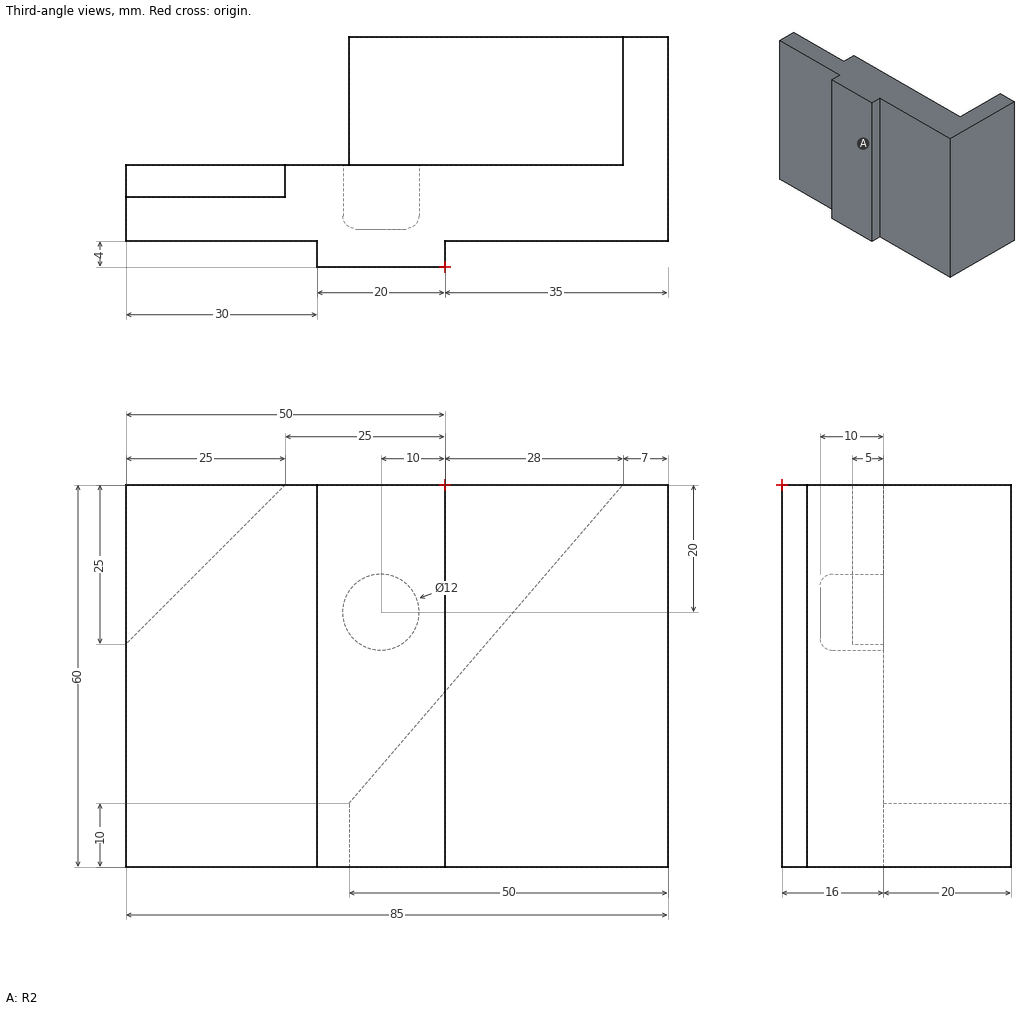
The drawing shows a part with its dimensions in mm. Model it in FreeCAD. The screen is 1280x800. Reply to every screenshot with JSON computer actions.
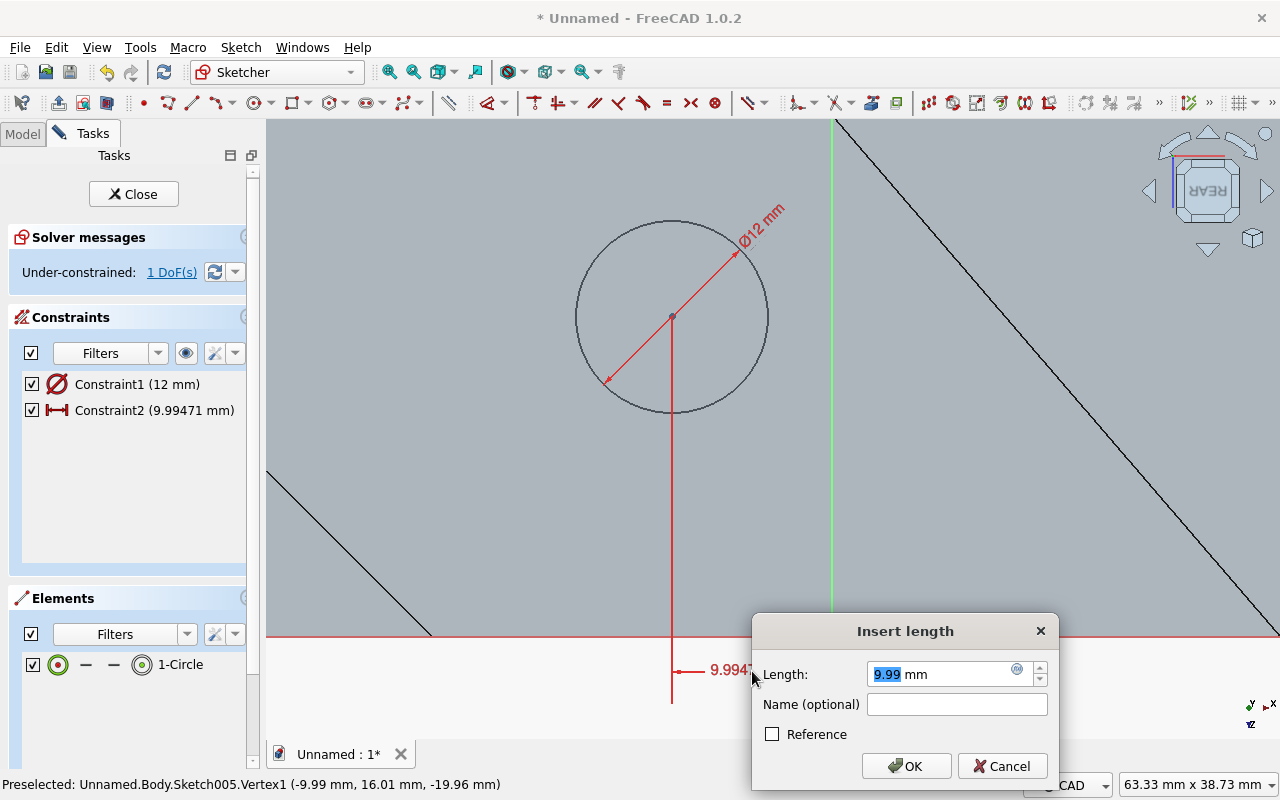
{"action": "type", "text": "10"}
{"action": "key", "text": "Return"}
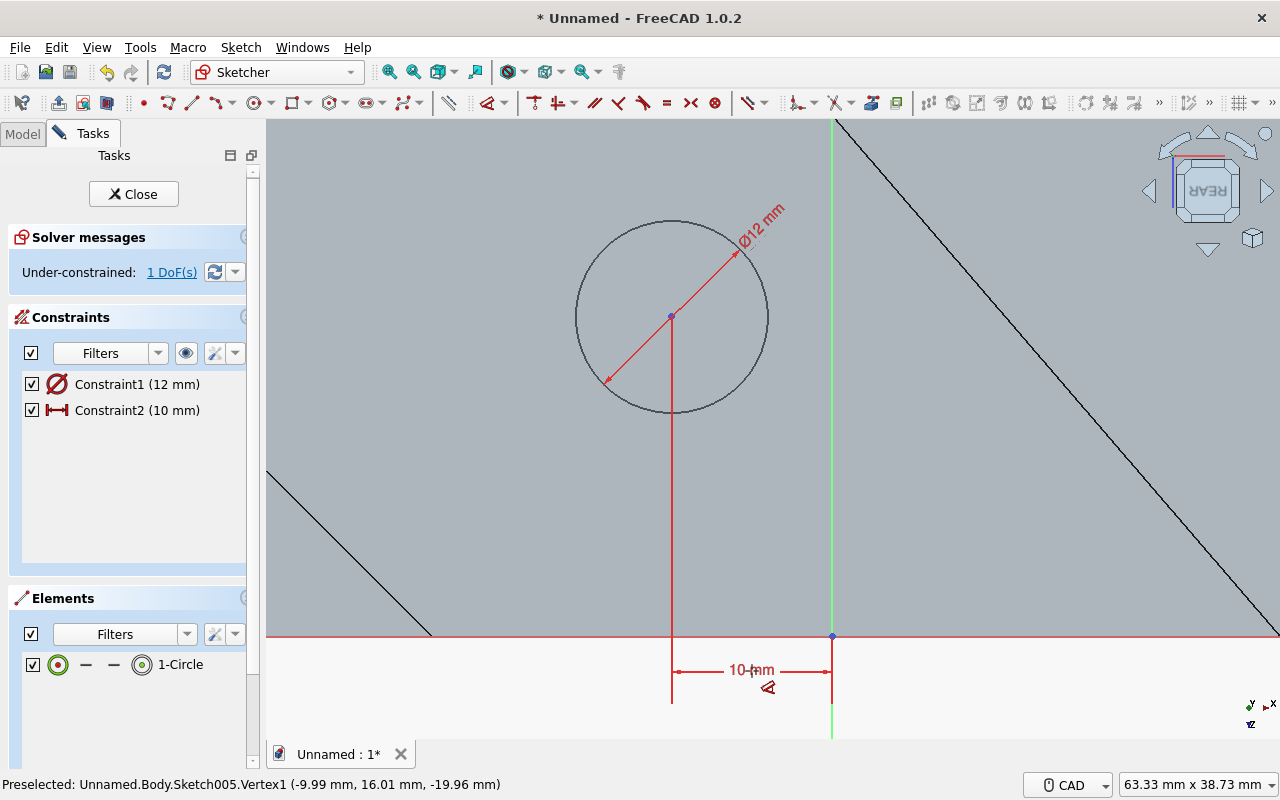
{"action": "left_click", "coordinate": [672, 317]}
{"action": "left_click", "coordinate": [866, 477]}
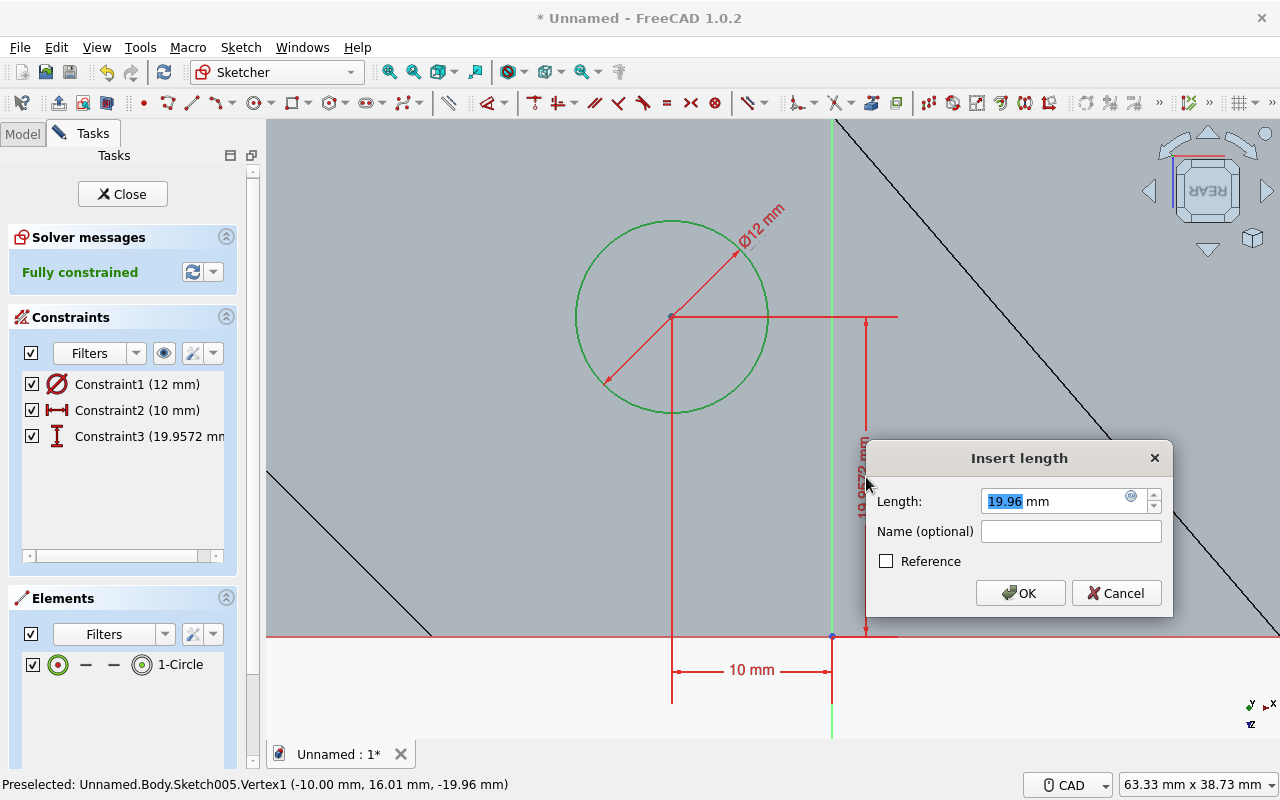
{"action": "type", "text": "20"}
{"action": "key", "text": "Return"}
{"action": "key", "text": "Escape"}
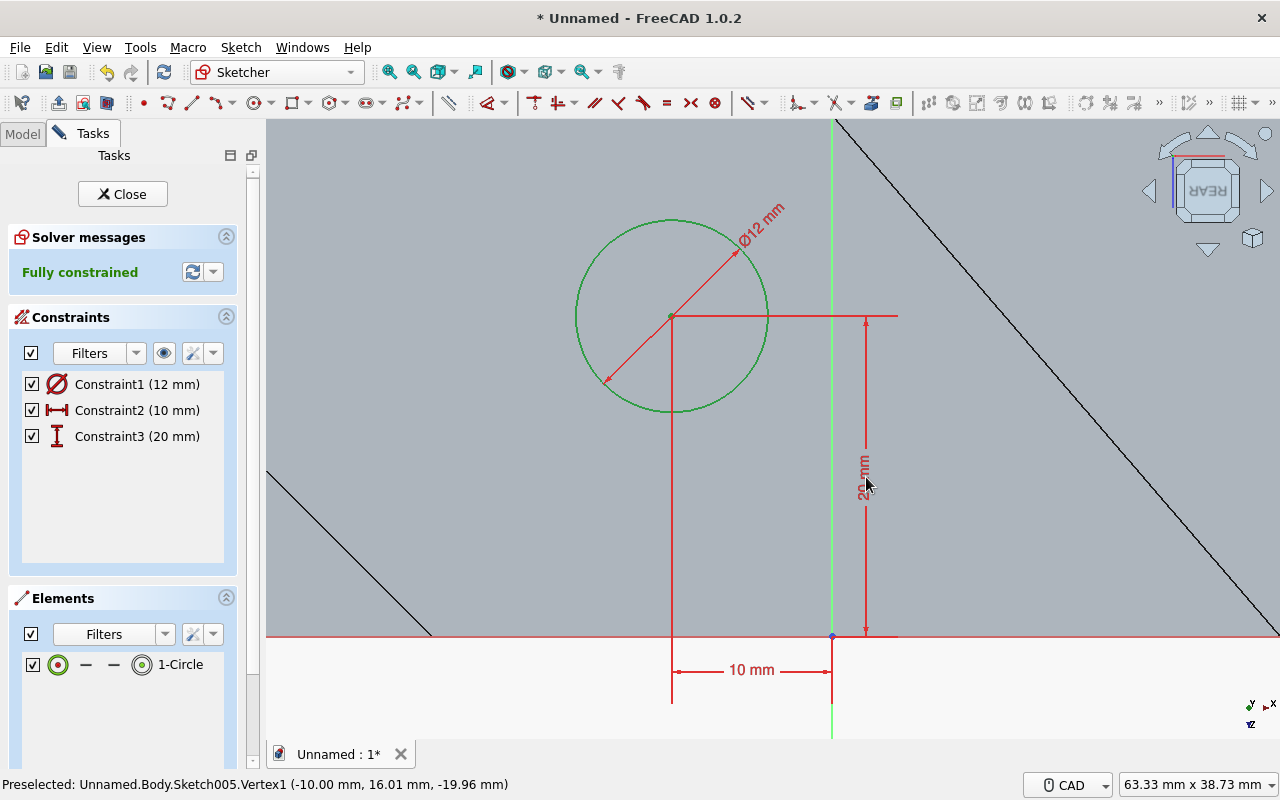
{"action": "left_click", "coordinate": [123, 194]}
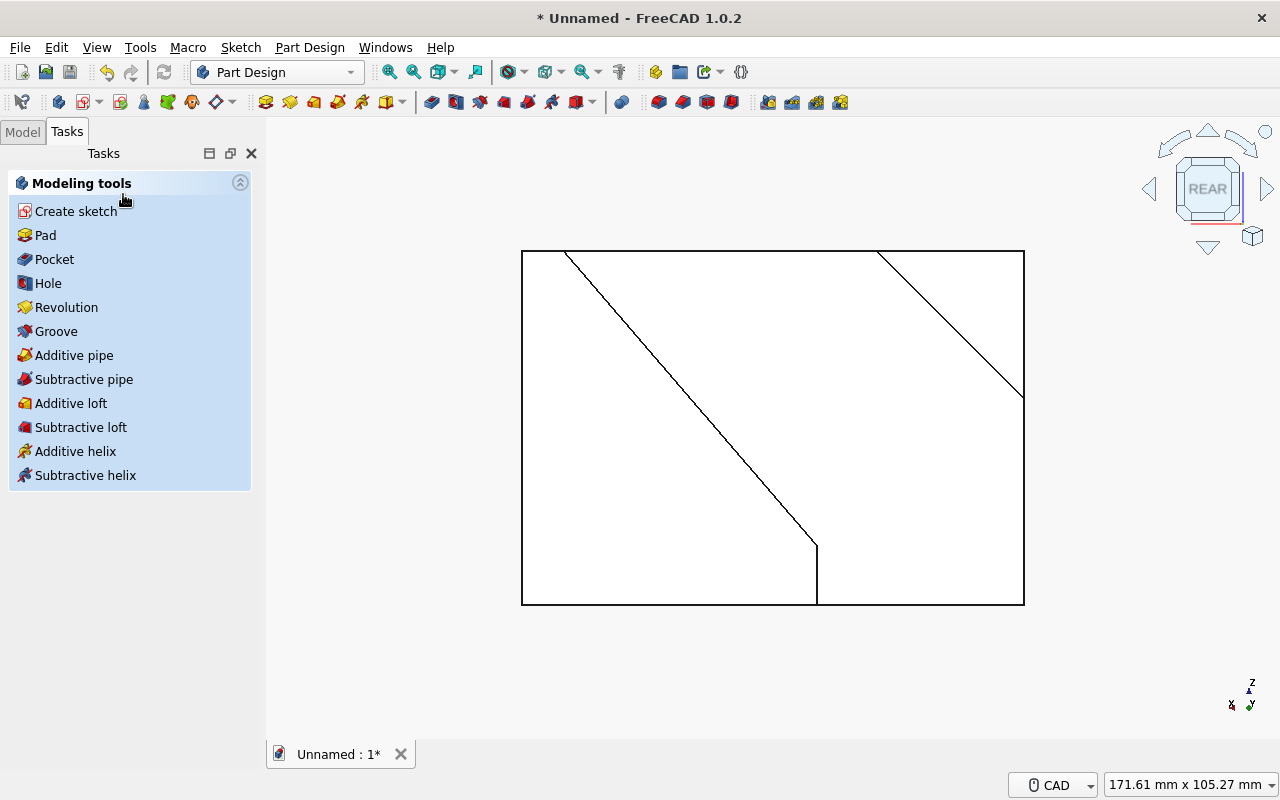
{"action": "left_click", "coordinate": [432, 102]}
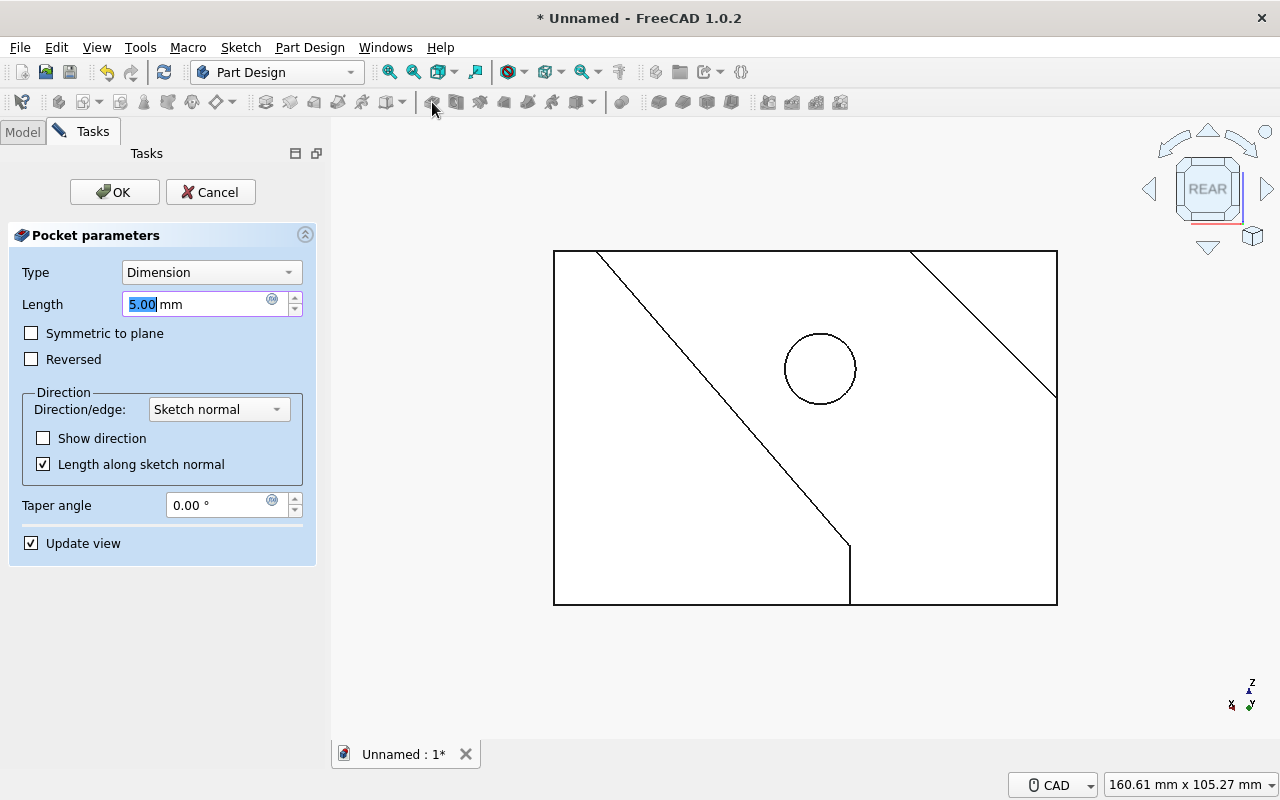
{"action": "type", "text": "10"}
{"action": "key", "text": "Tab"}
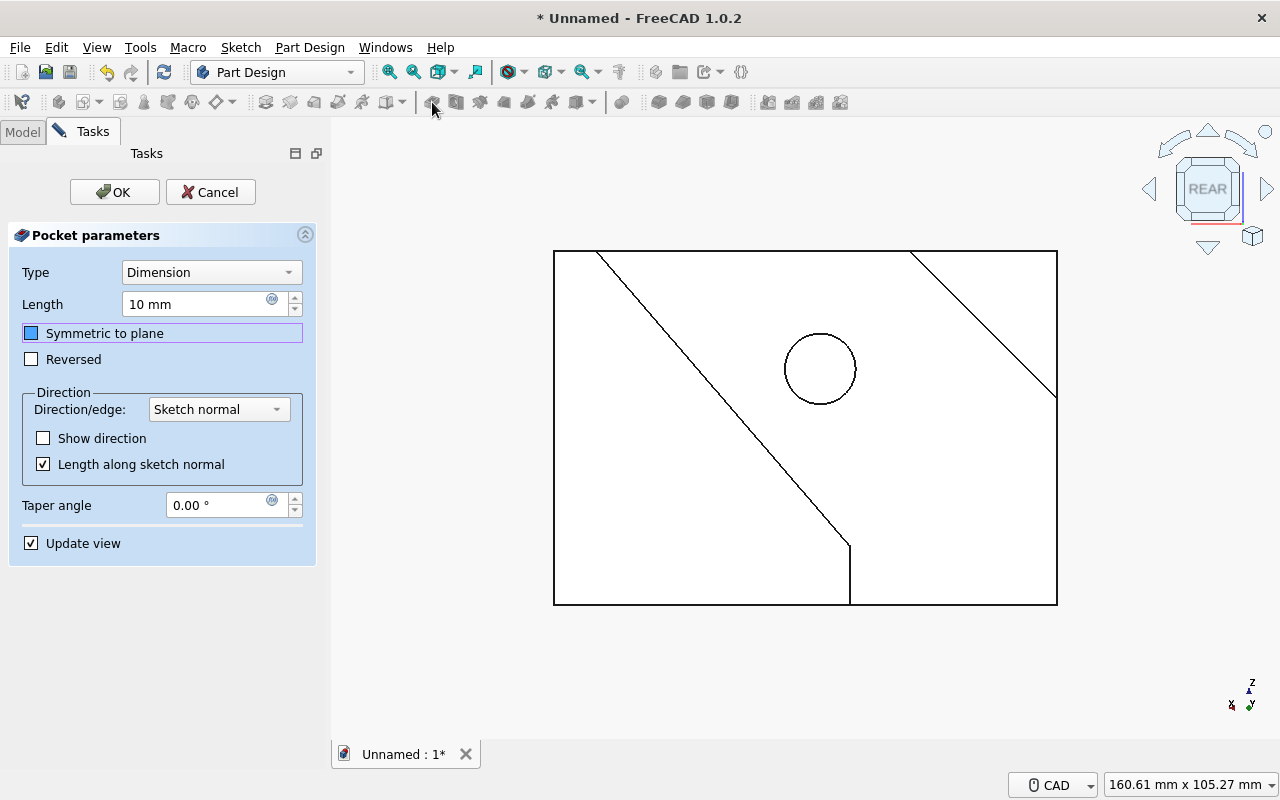
{"action": "left_click", "coordinate": [115, 192]}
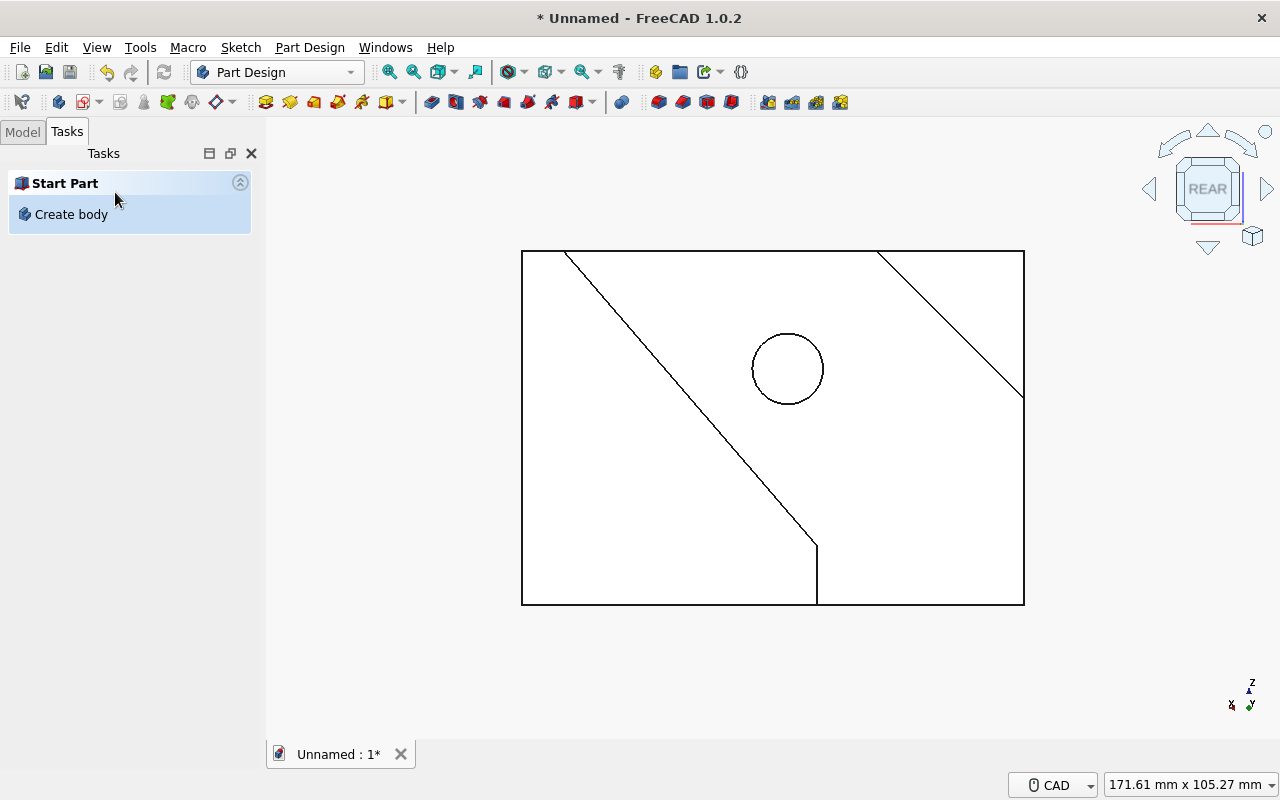
{"action": "key", "text": "0"}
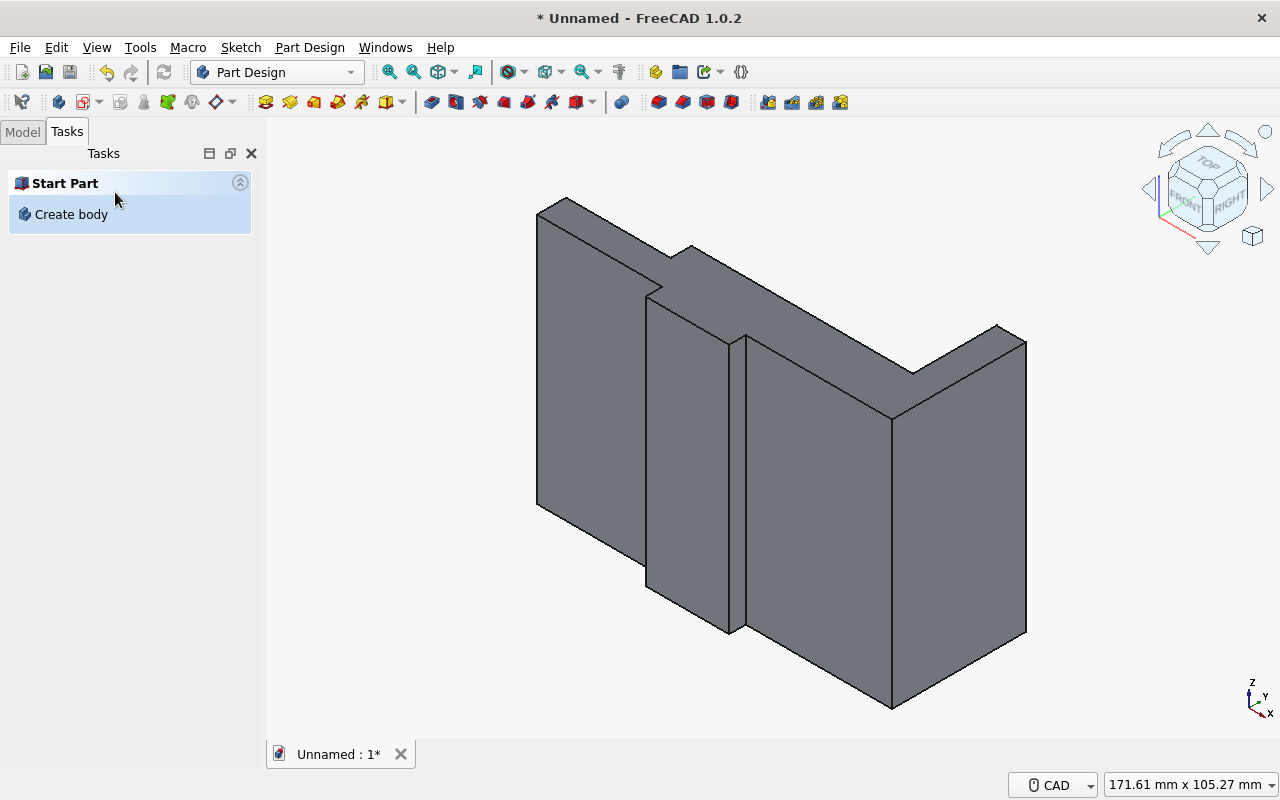
{"action": "key", "text": "2"}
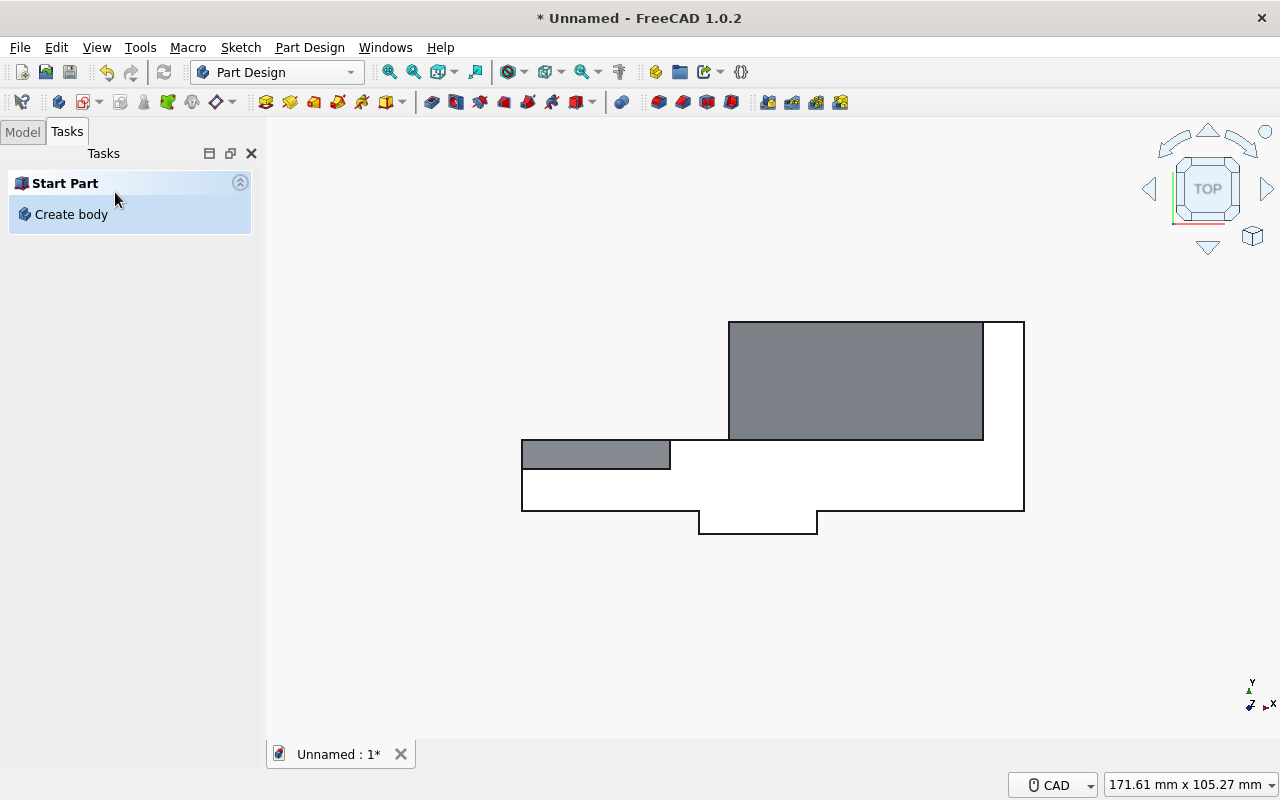
{"action": "key", "text": "1"}